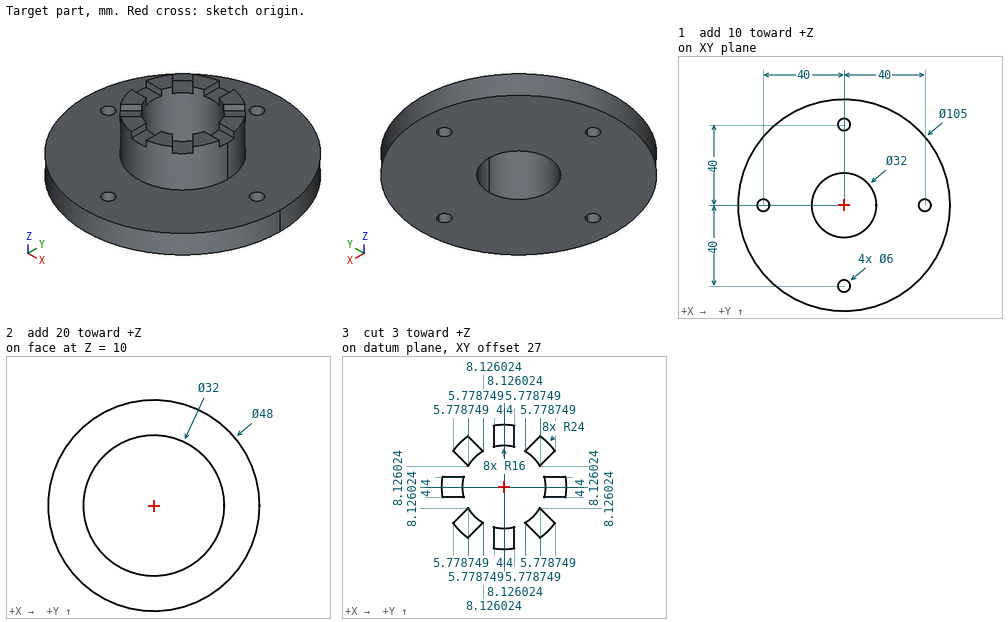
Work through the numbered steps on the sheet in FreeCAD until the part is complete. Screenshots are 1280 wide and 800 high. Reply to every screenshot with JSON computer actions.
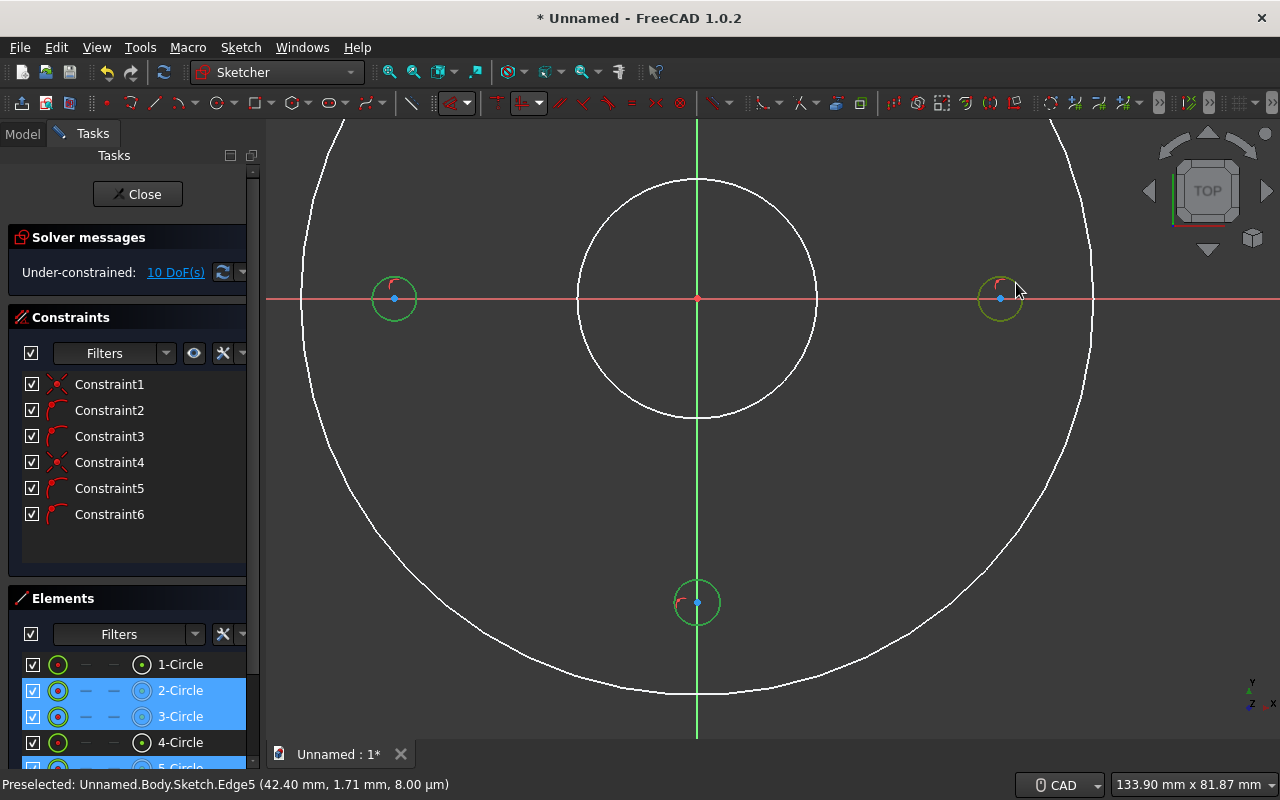
{"action": "scroll", "coordinate": [713, 587], "scroll_direction": "down", "scroll_amount": 3}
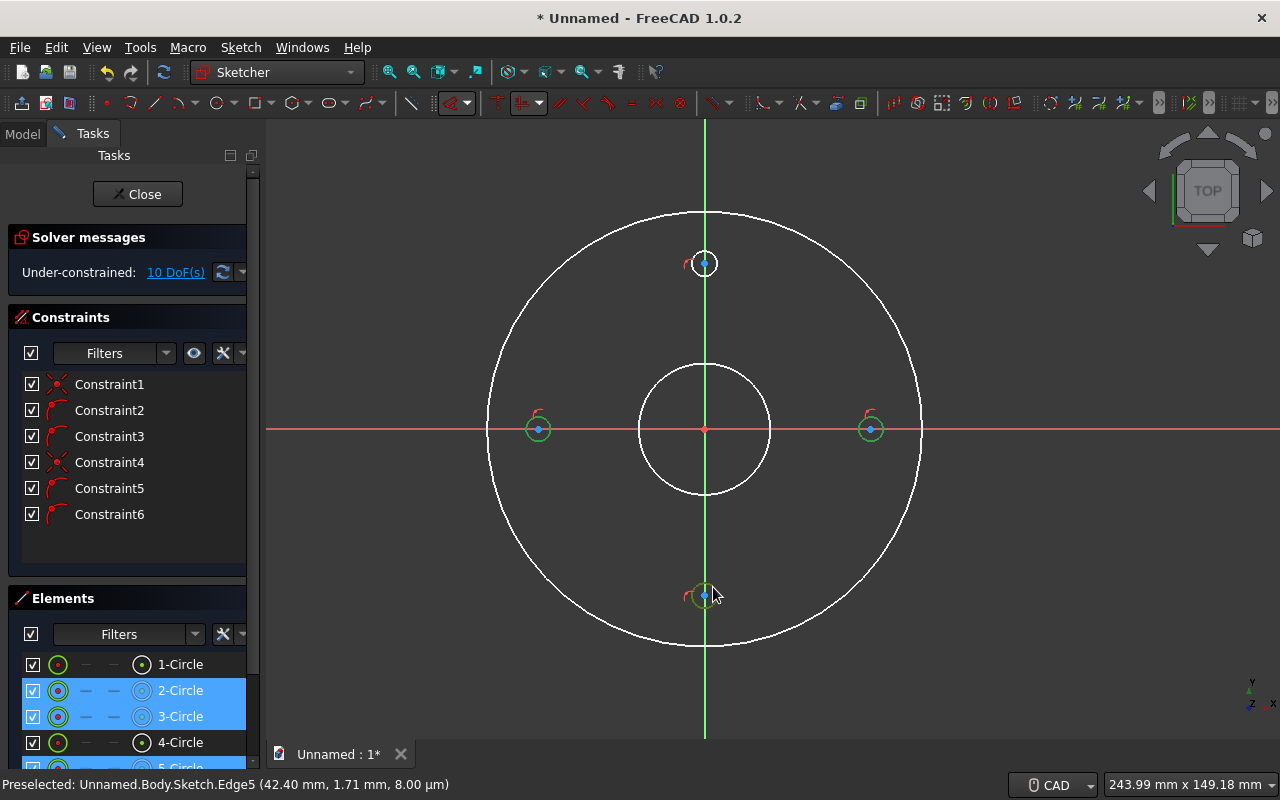
{"action": "scroll", "coordinate": [713, 255], "scroll_direction": "up", "scroll_amount": 3}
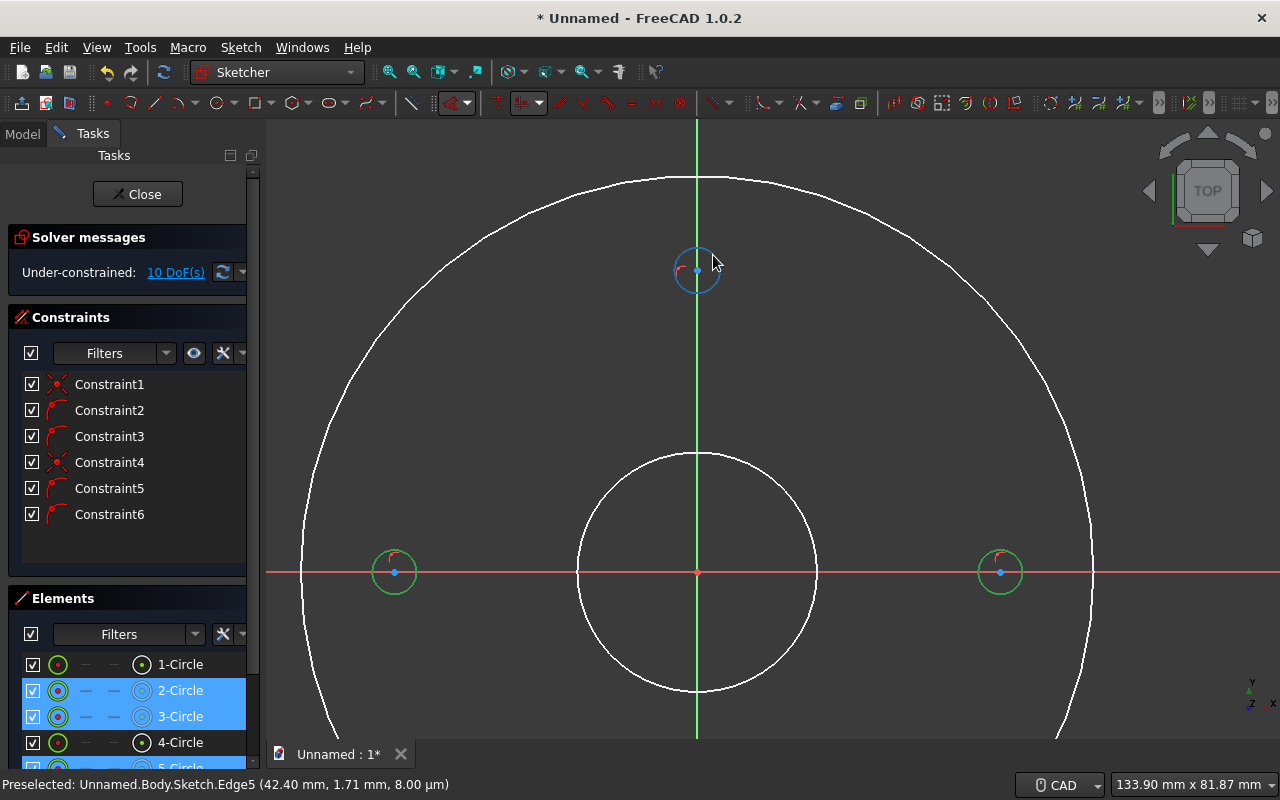
{"action": "left_click", "coordinate": [713, 254]}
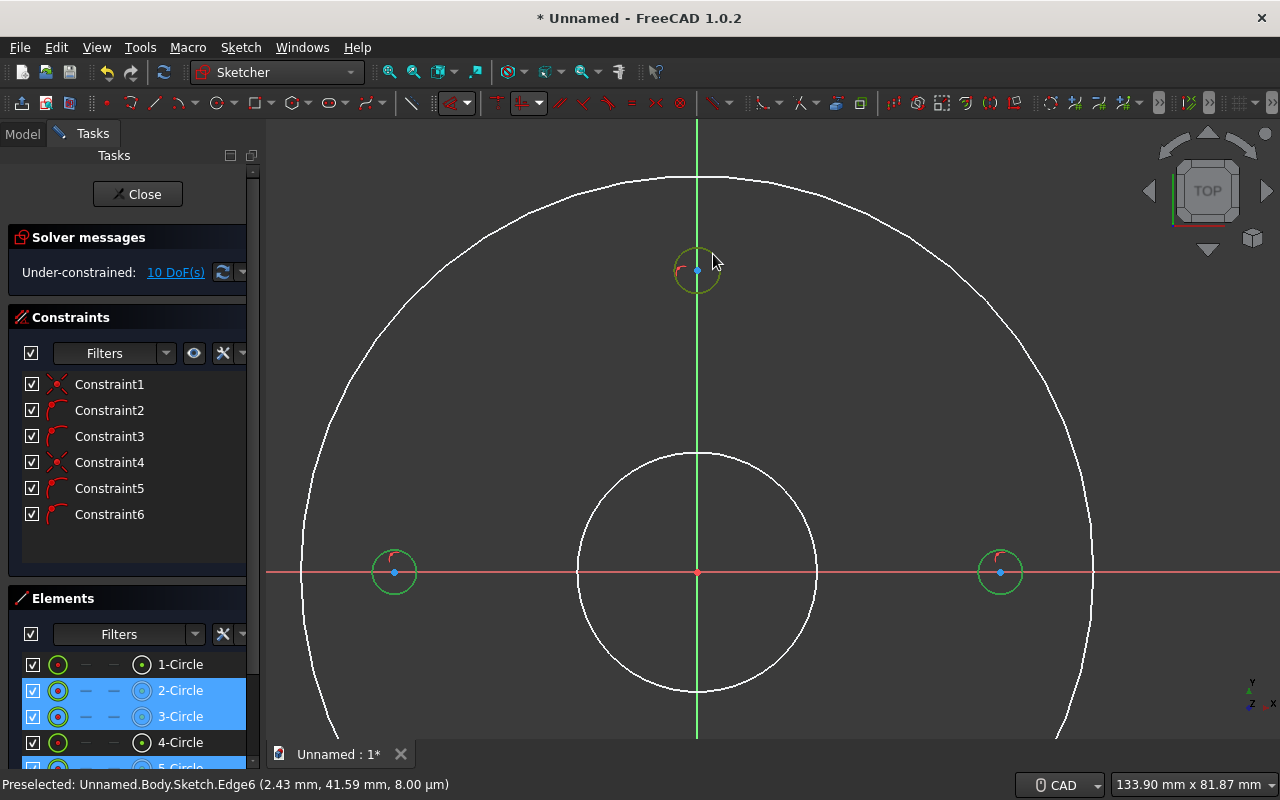
{"action": "left_click", "coordinate": [632, 104]}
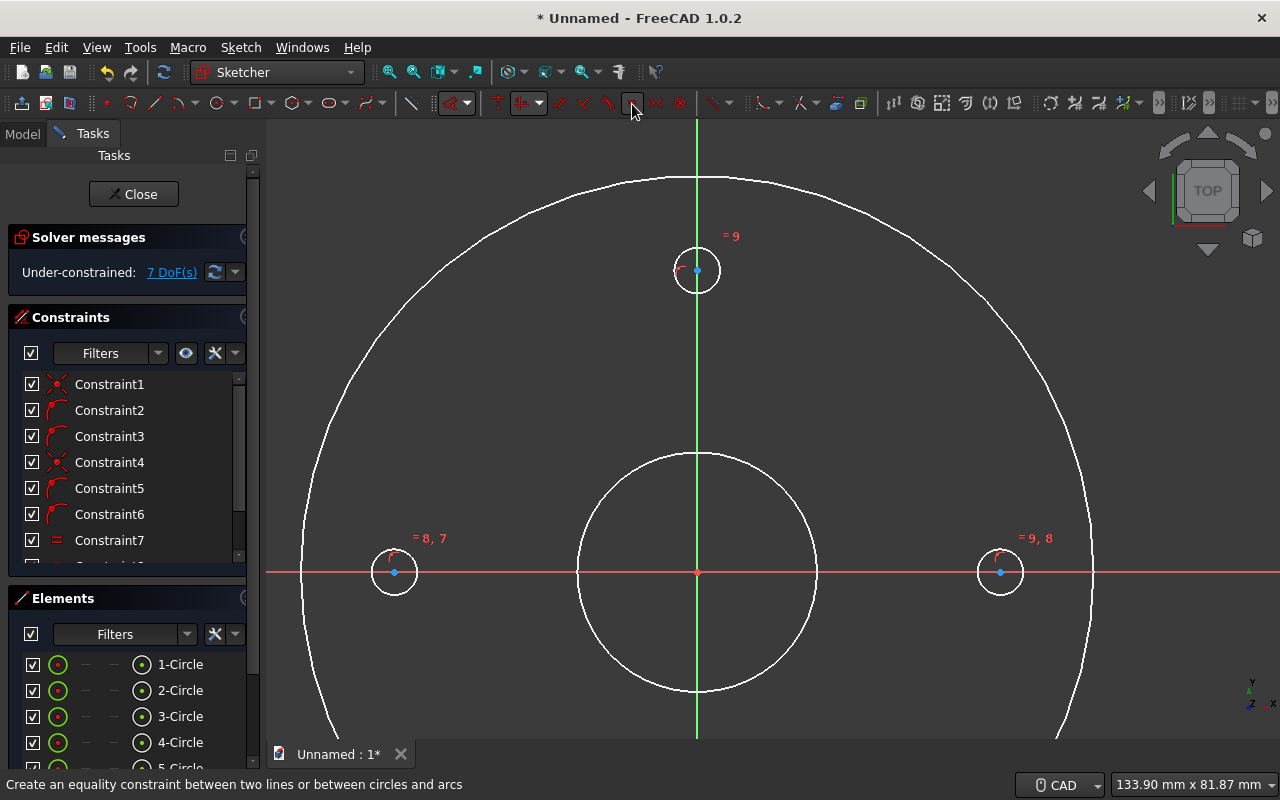
{"action": "left_click", "coordinate": [977, 291]}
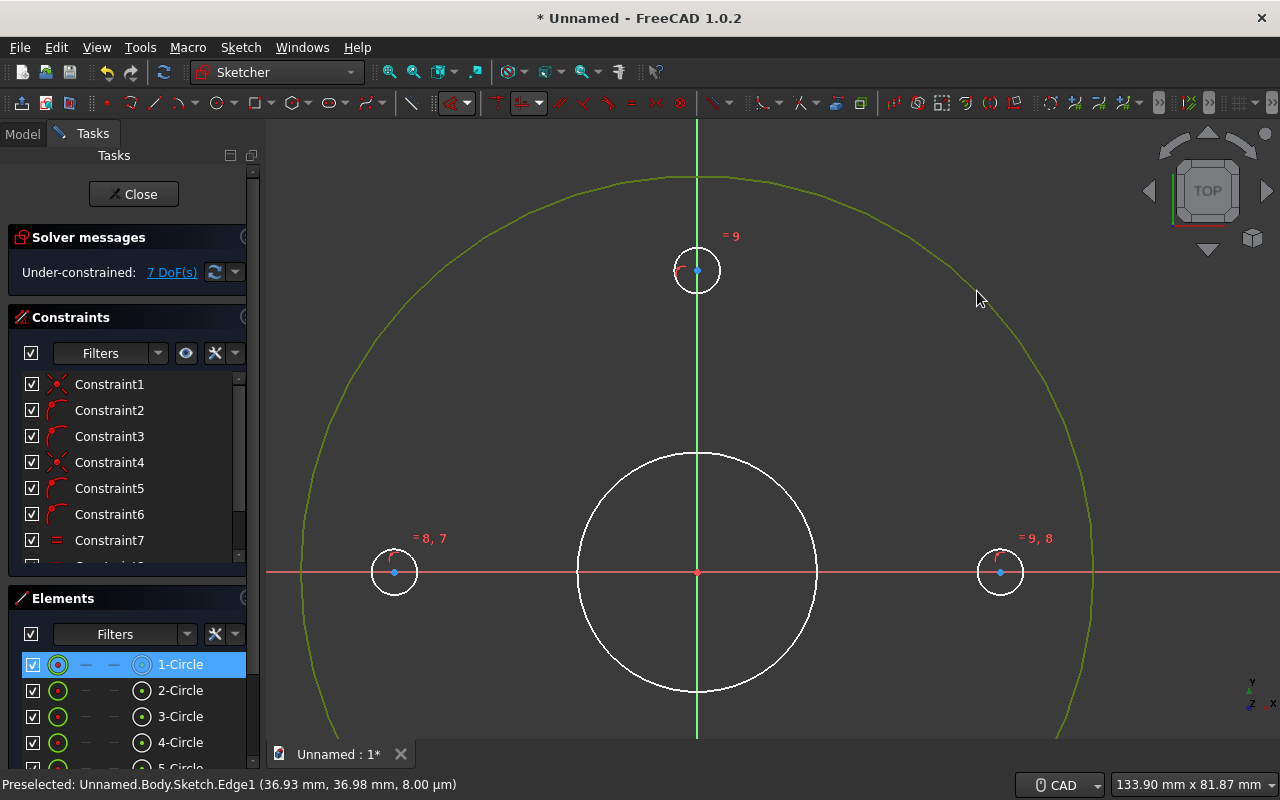
{"action": "left_click", "coordinate": [470, 104]}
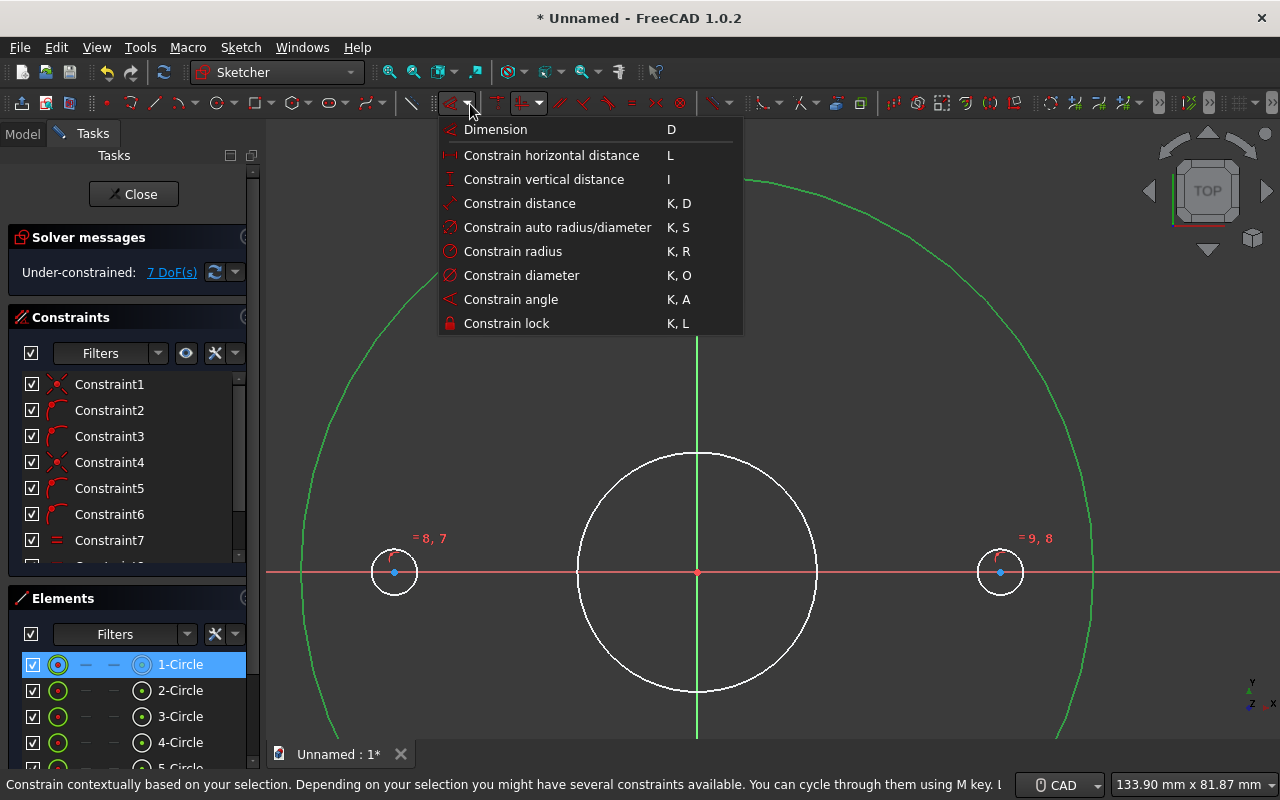
{"action": "left_click", "coordinate": [591, 275]}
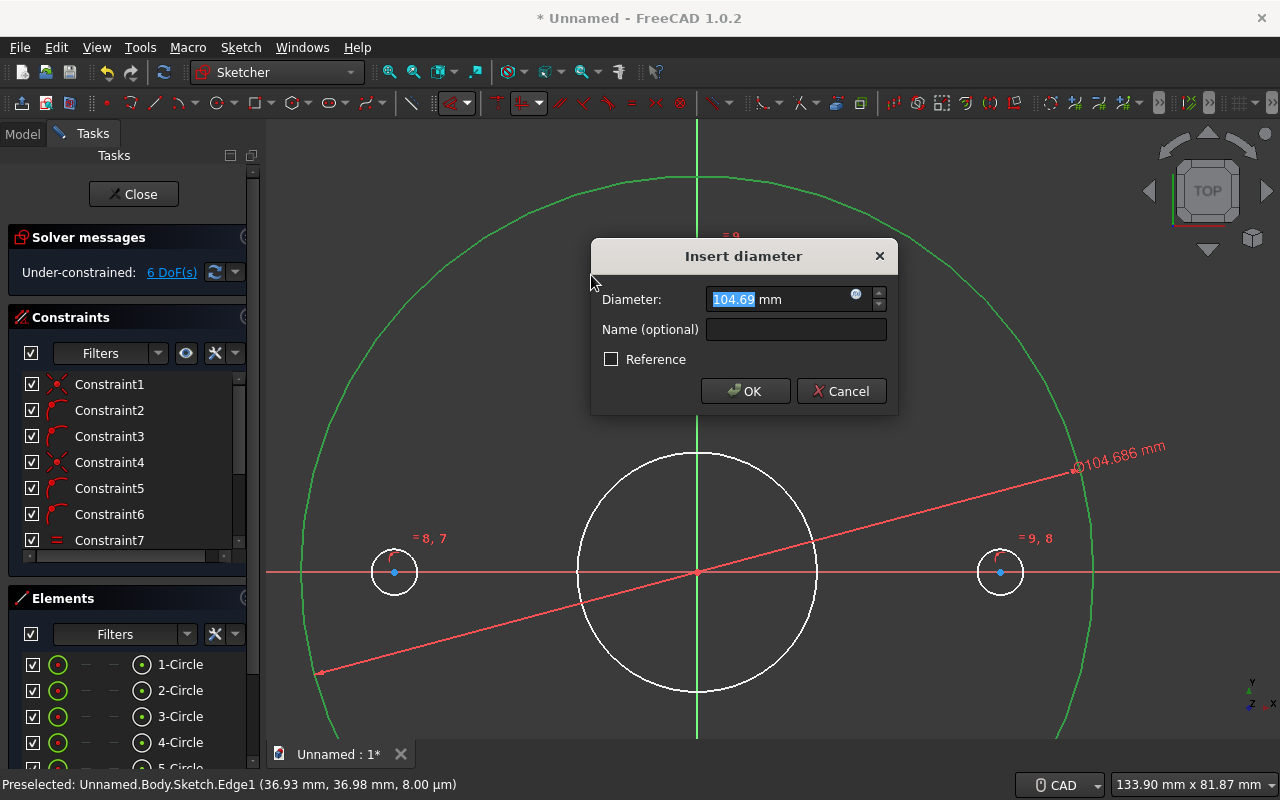
{"action": "type", "text": "105"}
{"action": "key", "text": "Return"}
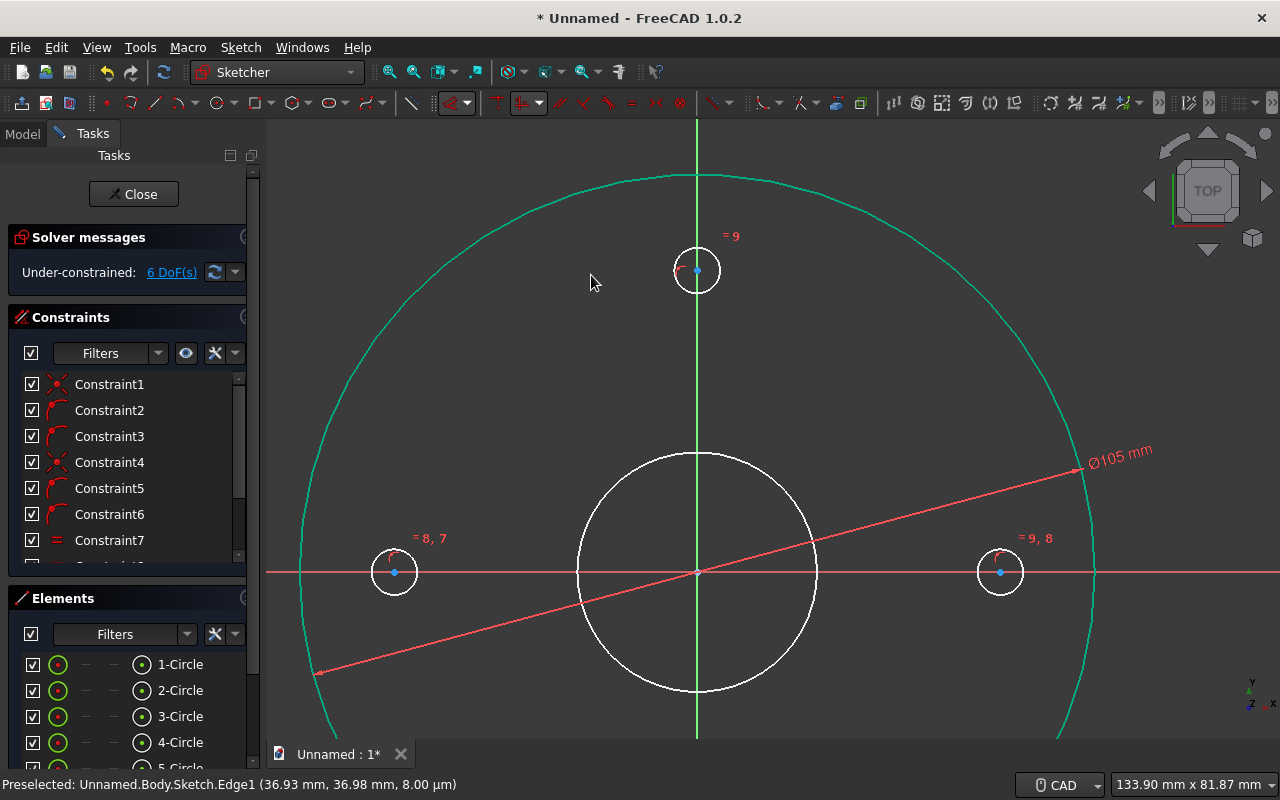
{"action": "scroll", "coordinate": [713, 255], "scroll_direction": "down", "scroll_amount": 3}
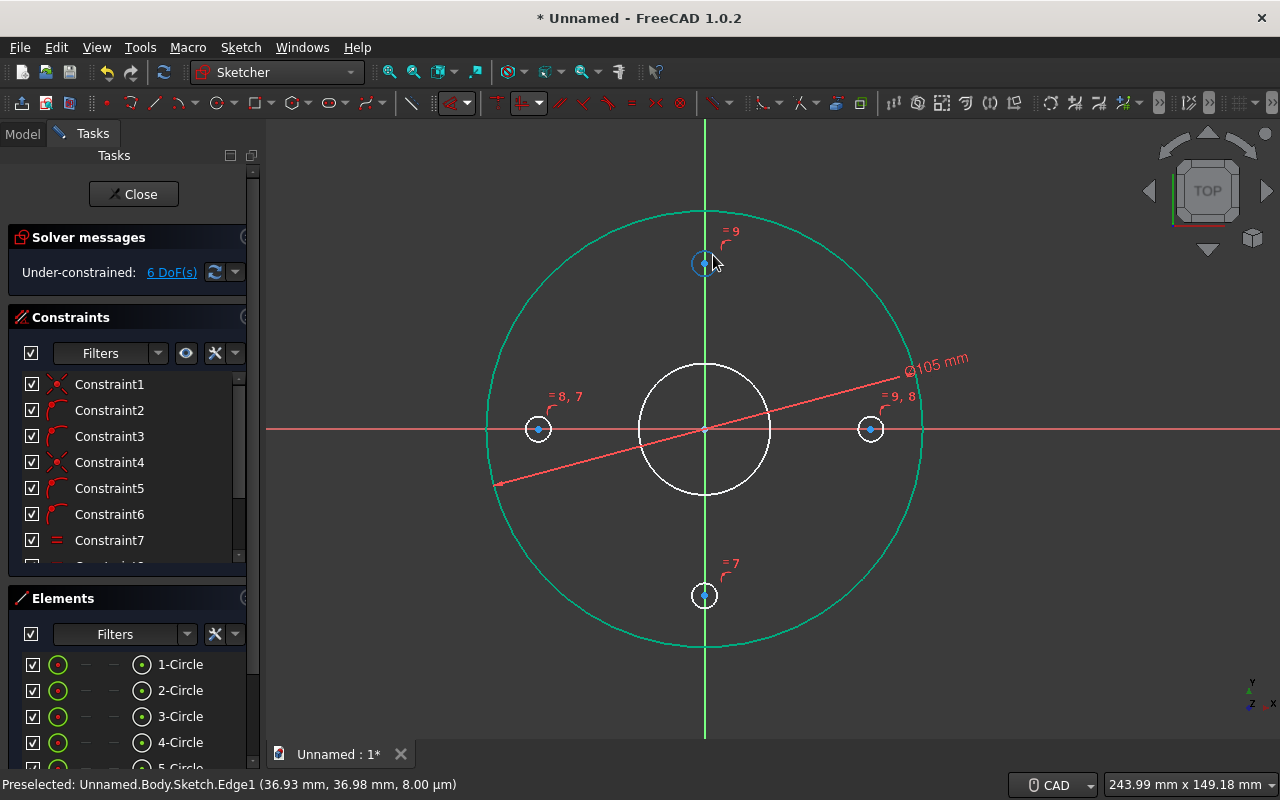
{"action": "scroll", "coordinate": [713, 587], "scroll_direction": "up", "scroll_amount": 3}